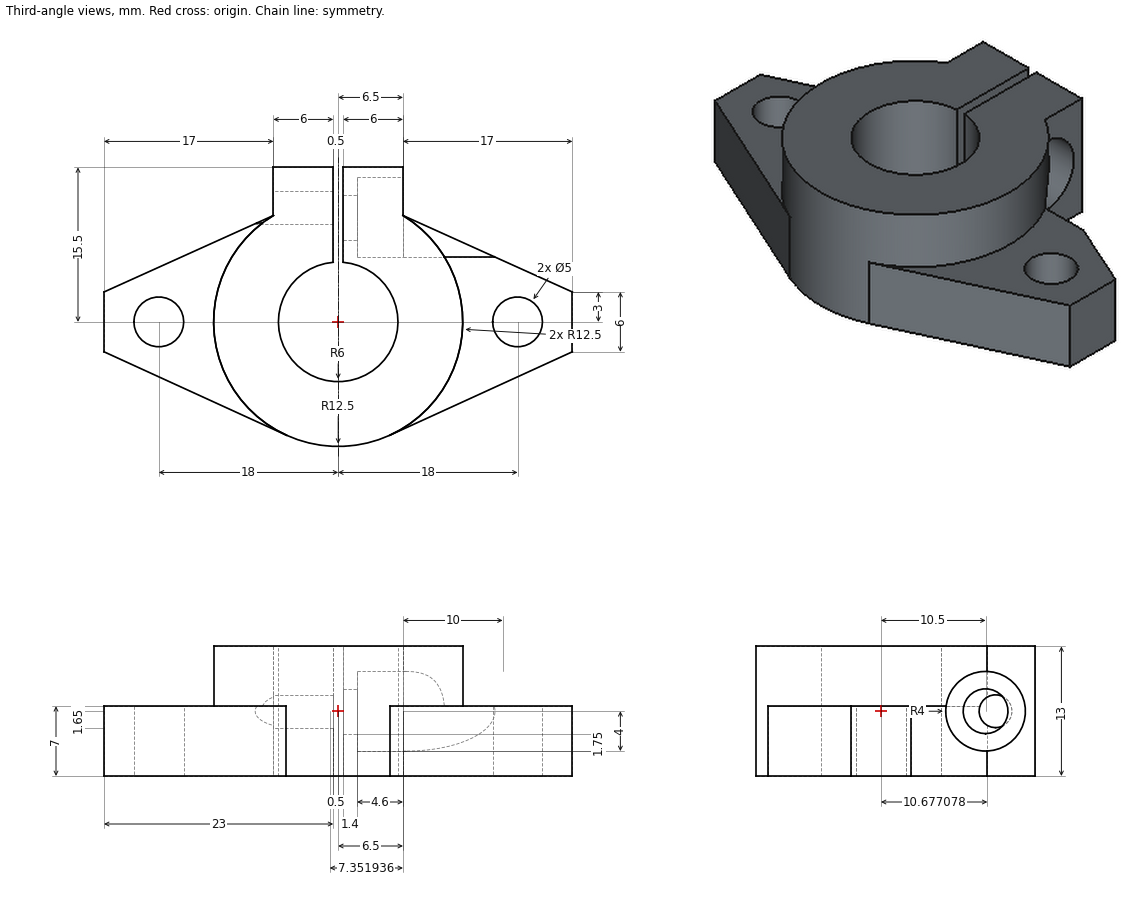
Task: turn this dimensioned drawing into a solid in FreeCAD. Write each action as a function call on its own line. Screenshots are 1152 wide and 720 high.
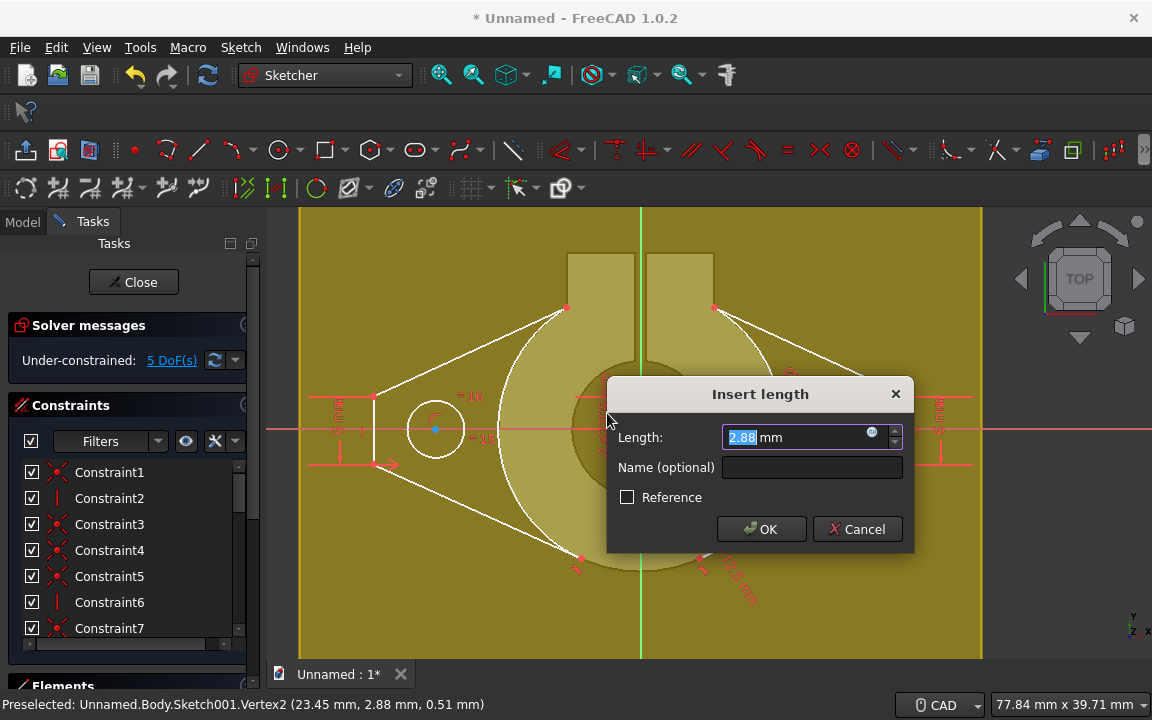
text(3)
key(Return)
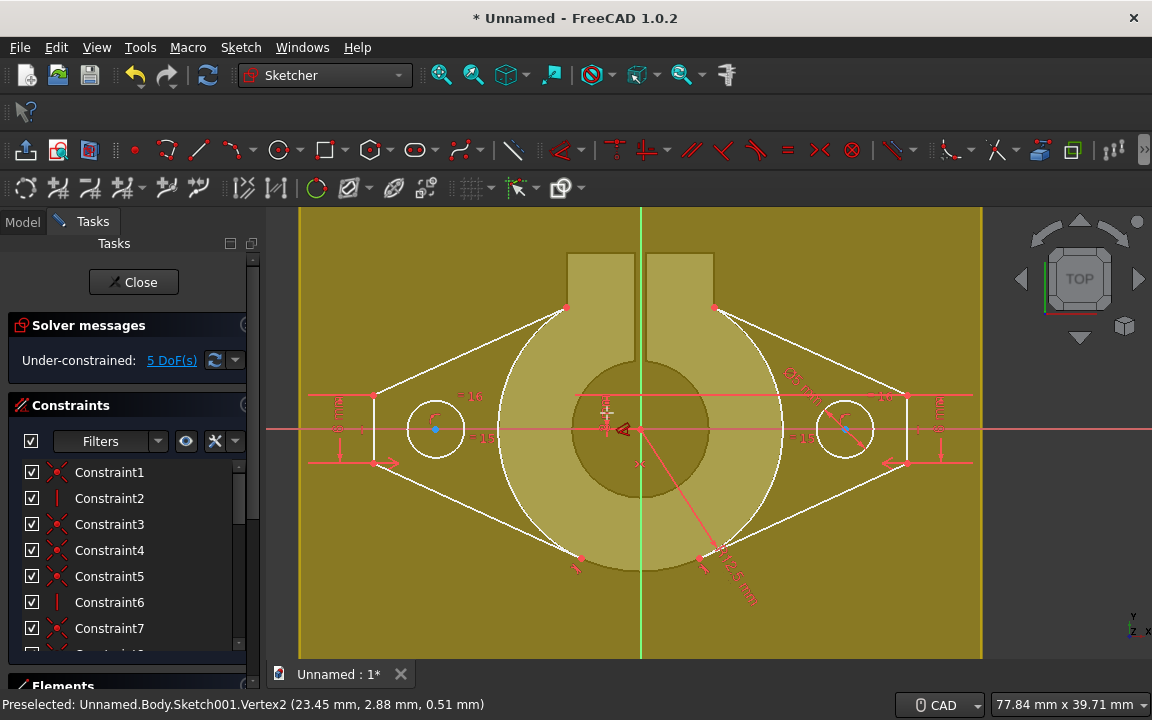
click(845, 429)
click(696, 395)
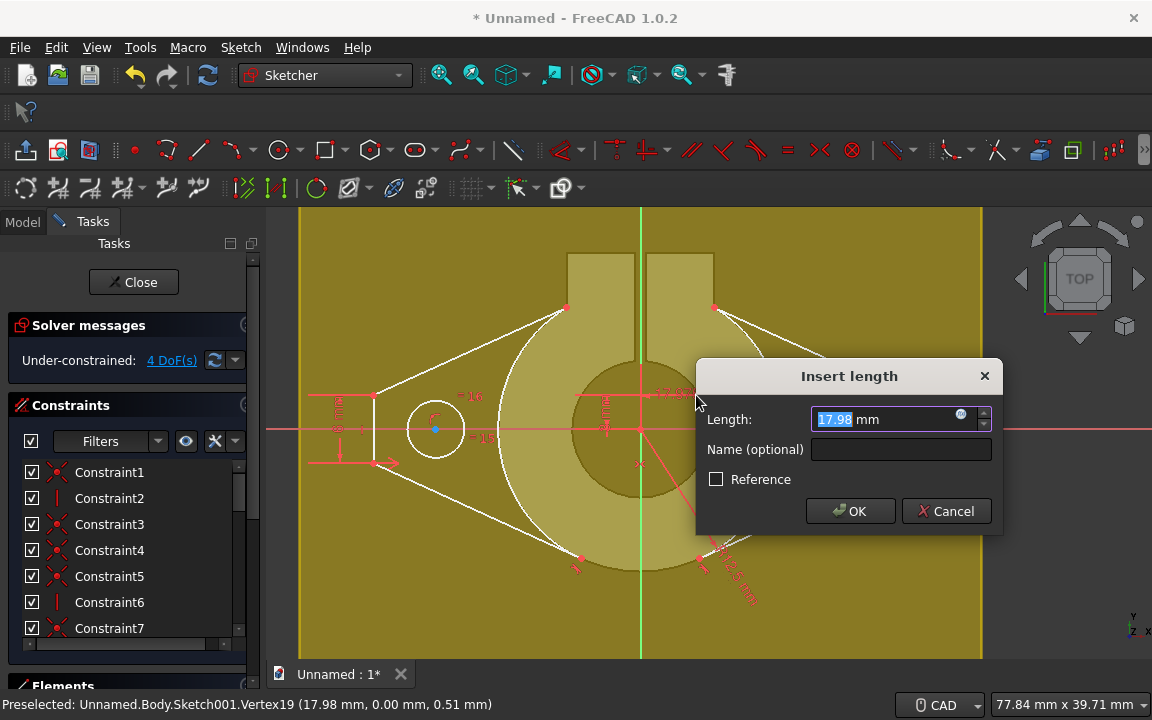
text(18)
key(Return)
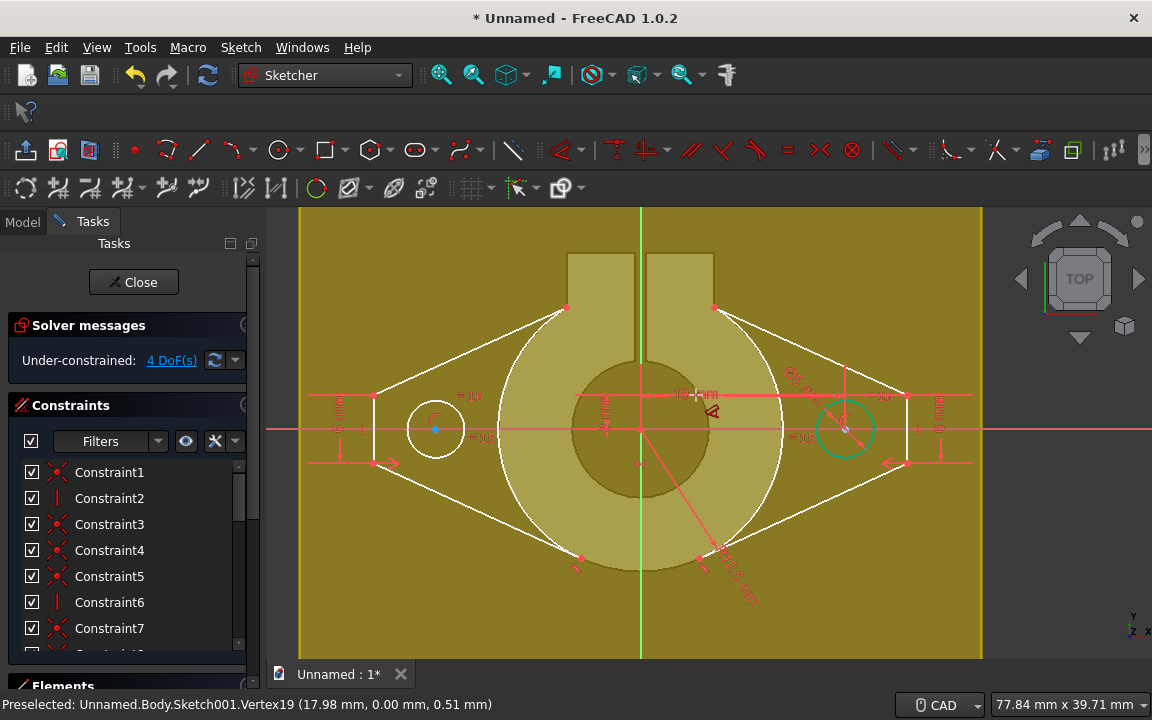
click(436, 429)
click(467, 395)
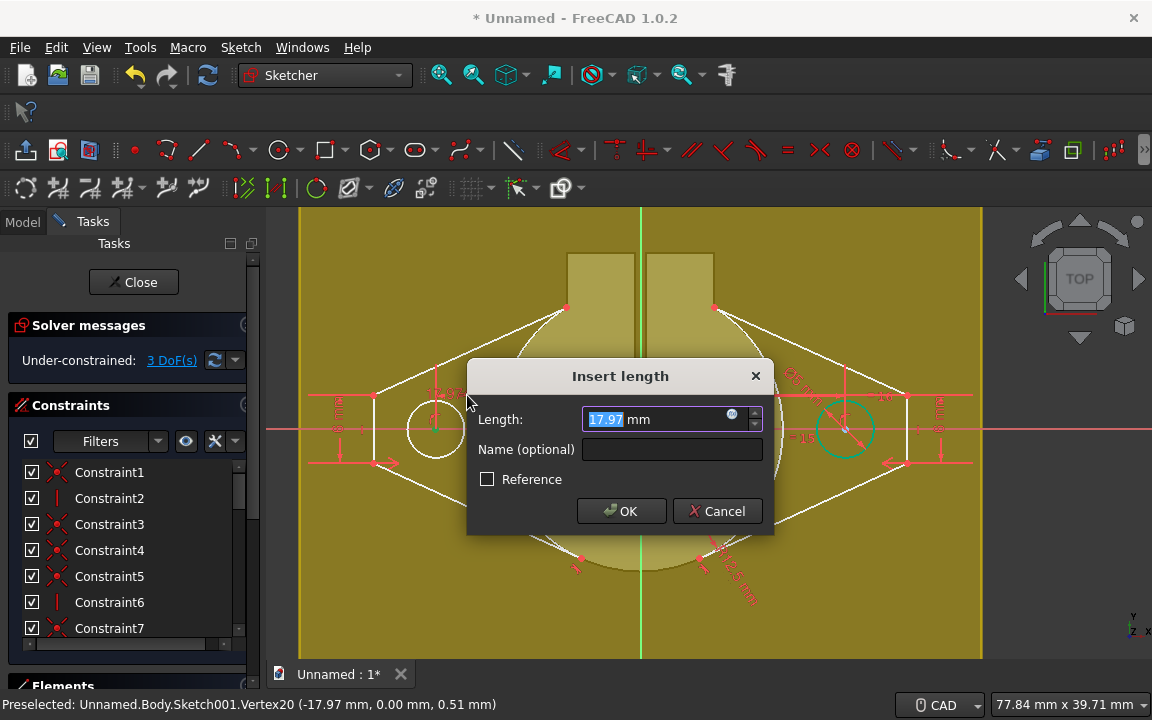
text(18)
key(Return)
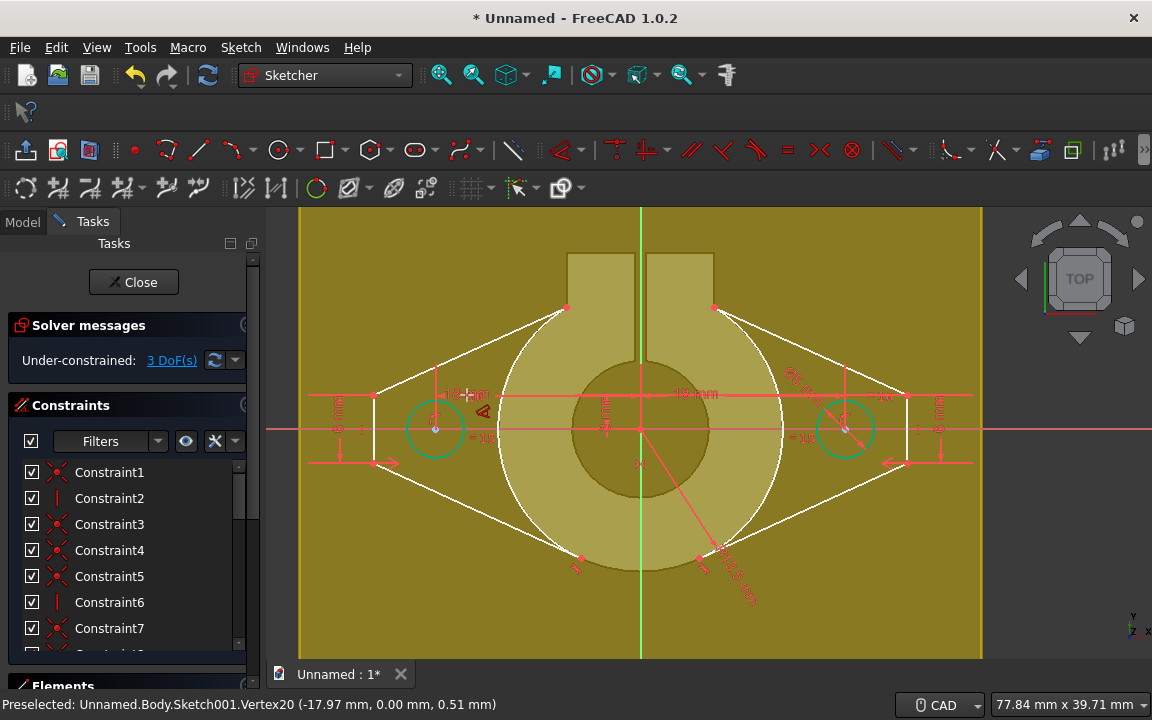
click(772, 334)
click(811, 274)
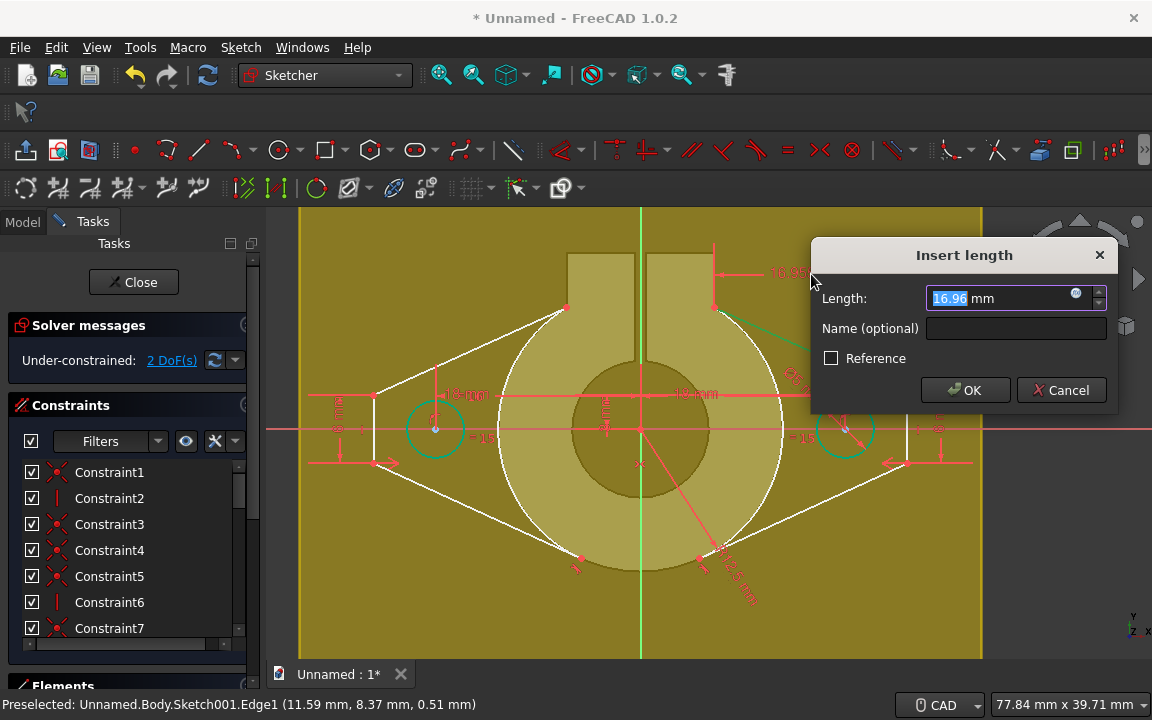
text(17)
key(Return)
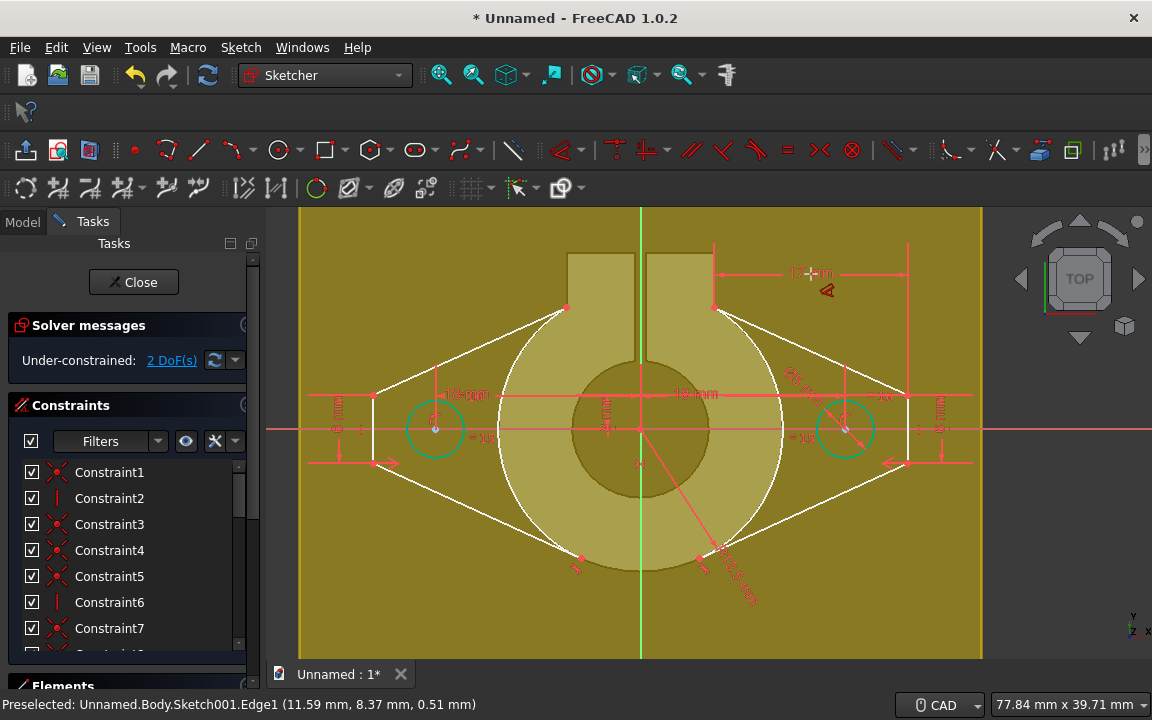
click(431, 369)
click(470, 274)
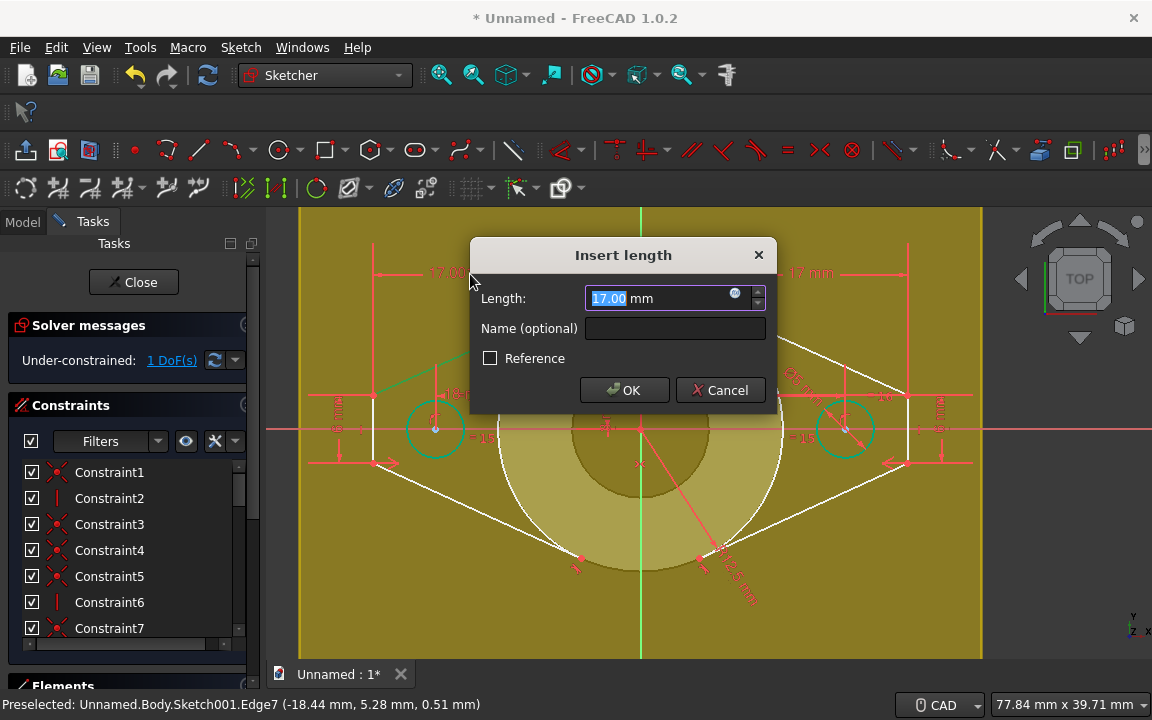
text(17)
key(Return)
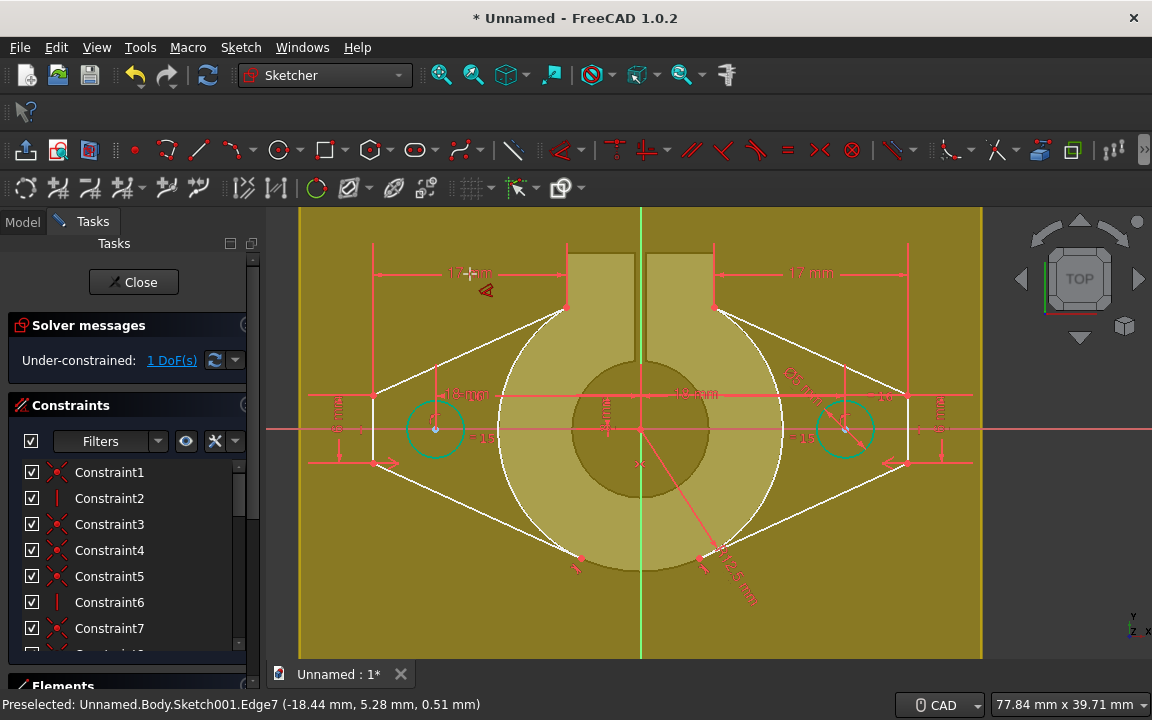
click(714, 308)
click(677, 274)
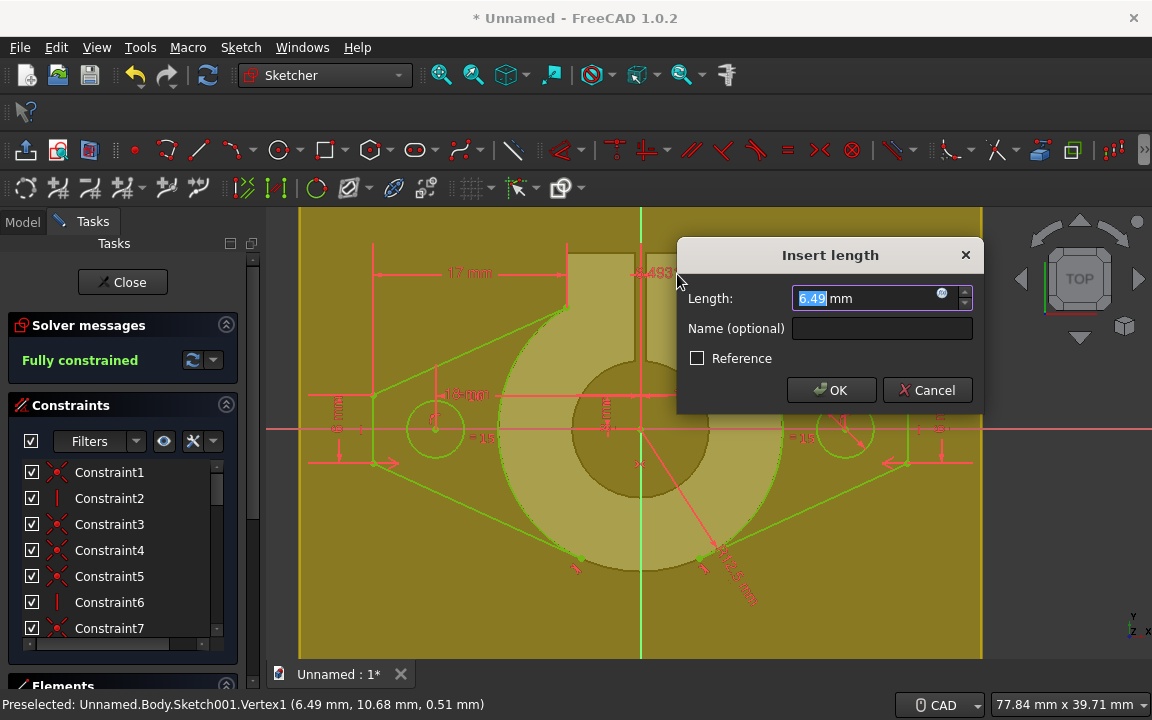
text(6.5)
key(Return)
key(Escape)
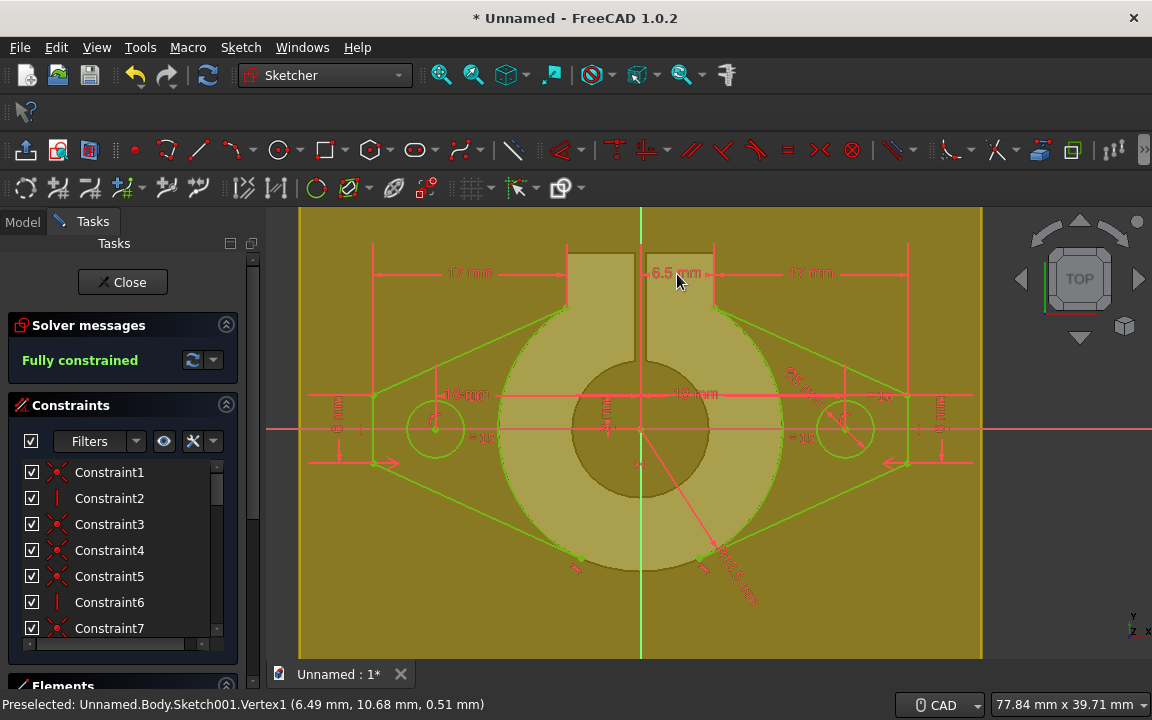
click(123, 282)